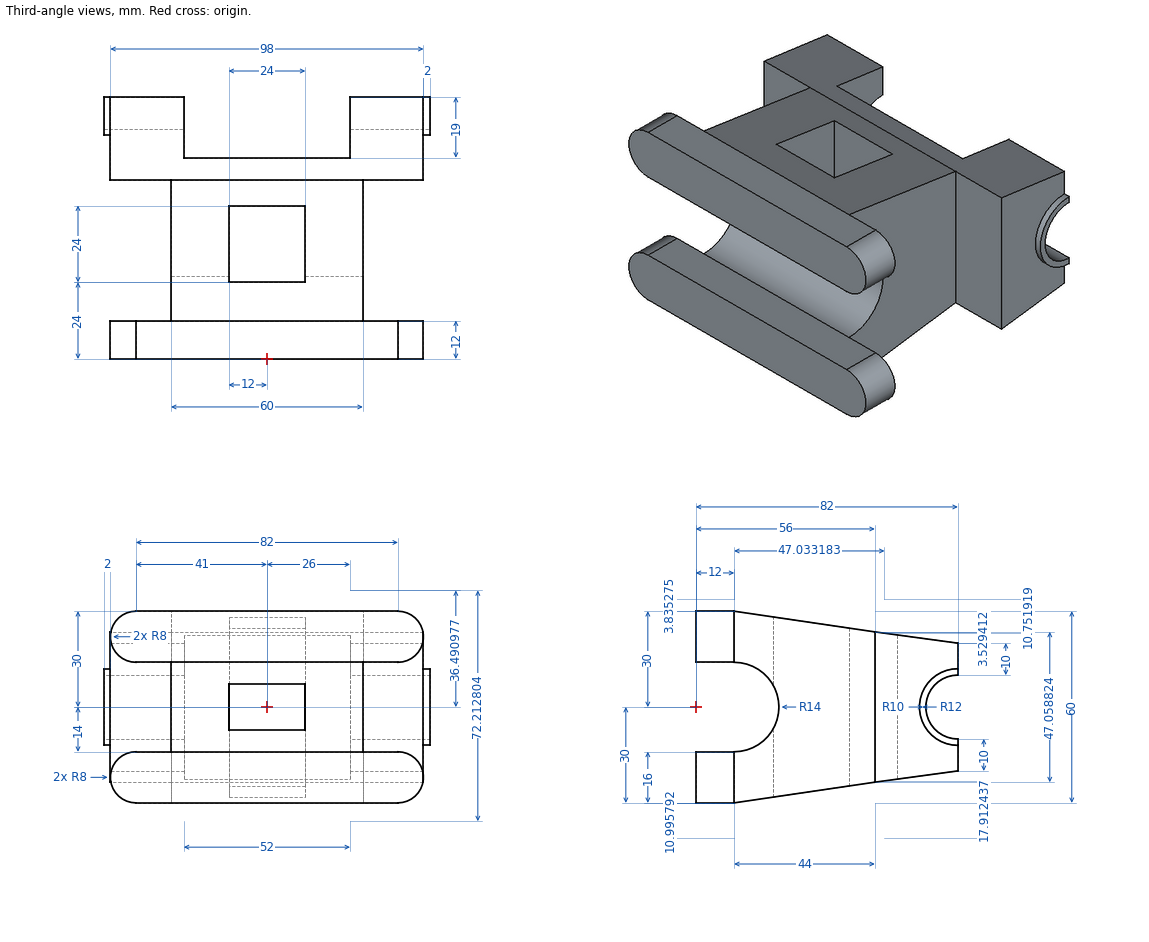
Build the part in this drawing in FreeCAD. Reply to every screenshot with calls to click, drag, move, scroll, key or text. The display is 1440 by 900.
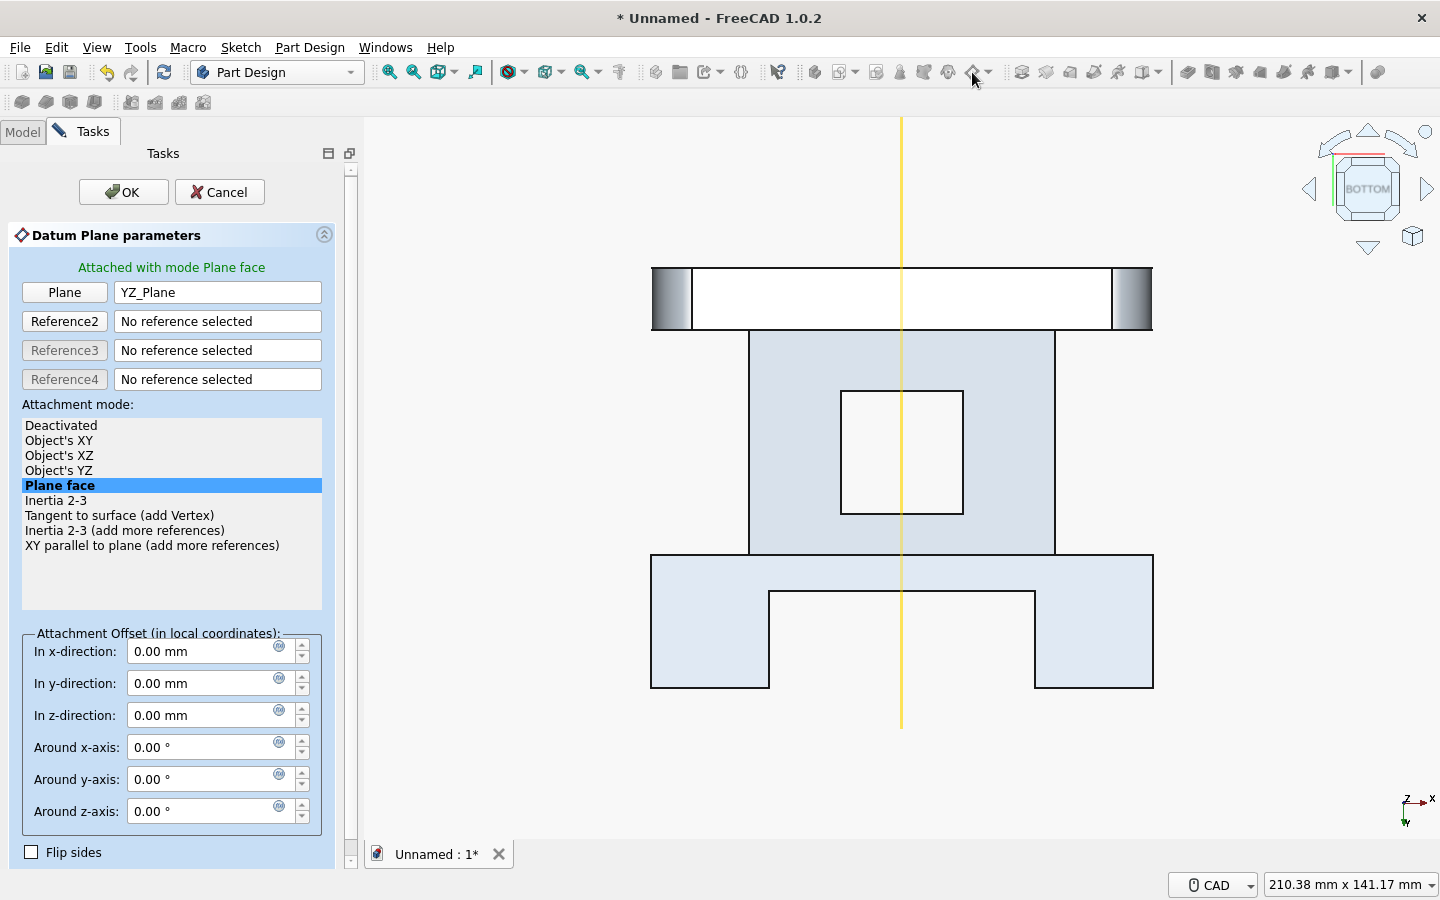
triple_click(210, 715)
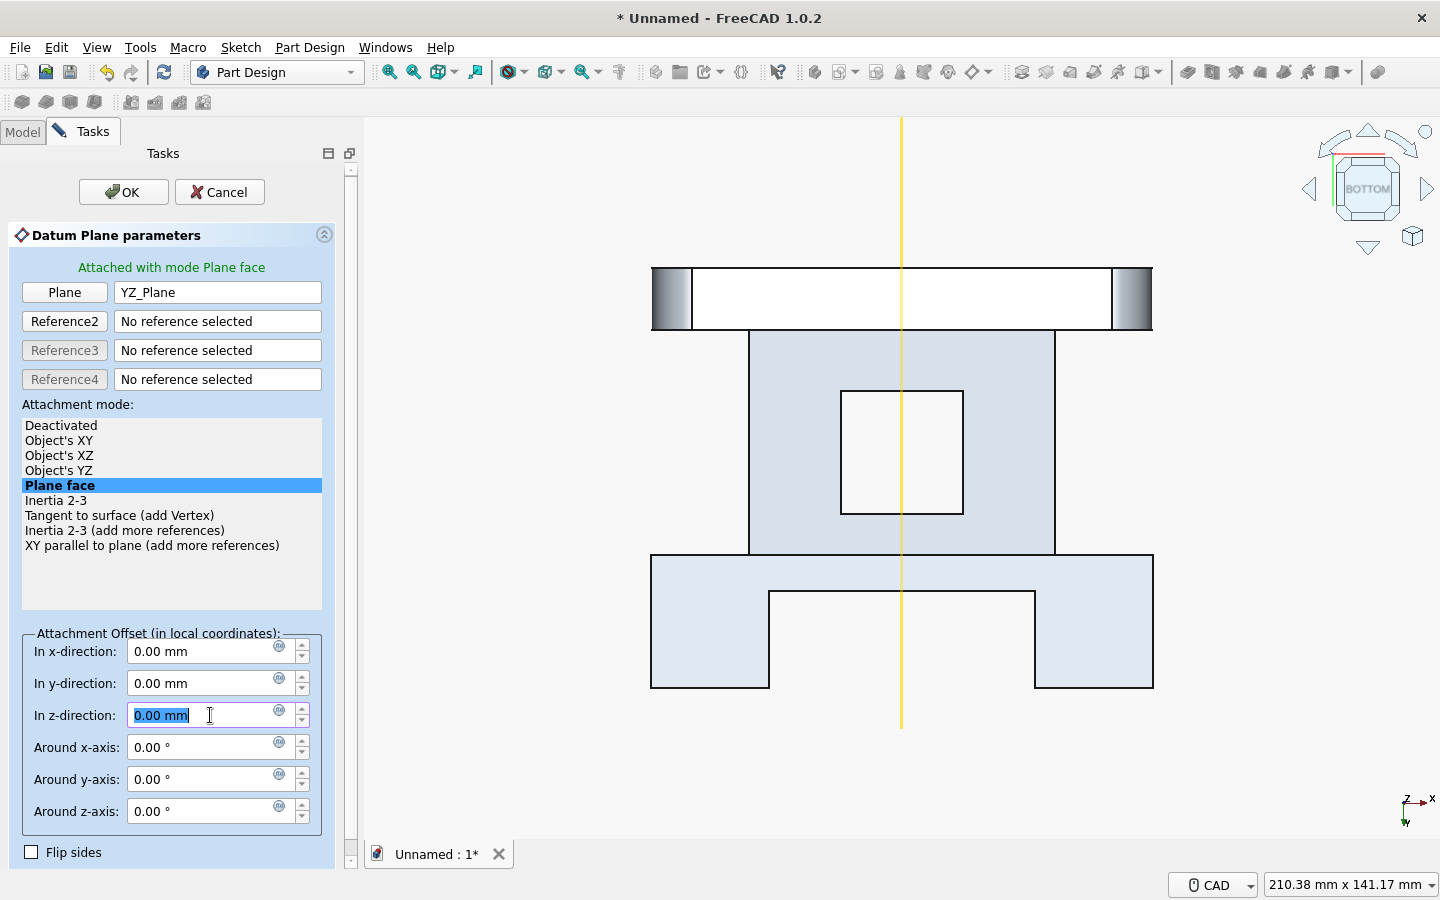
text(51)
key(Tab)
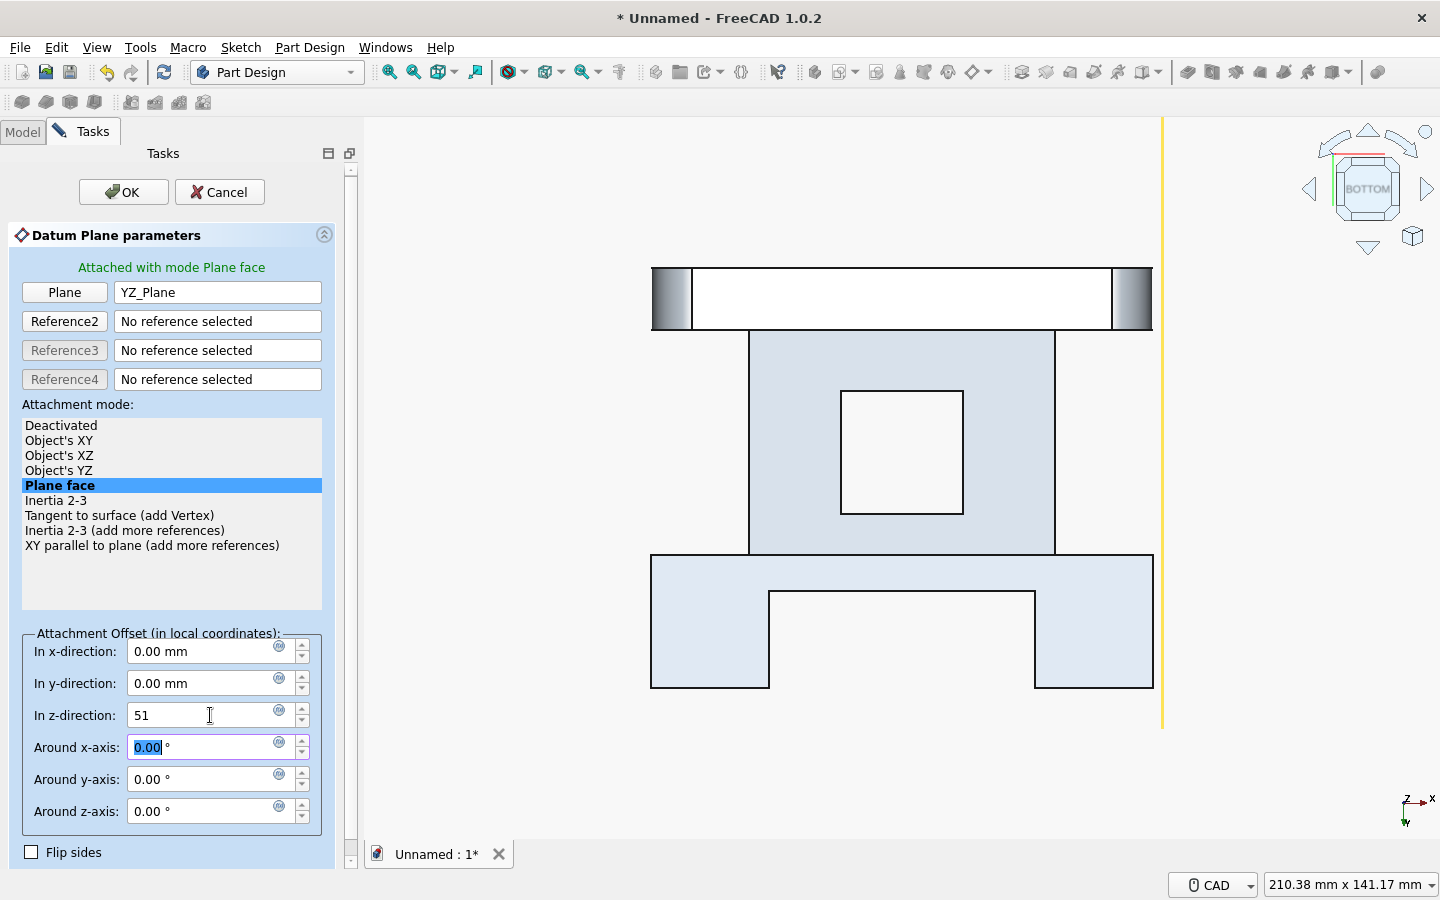
click(124, 192)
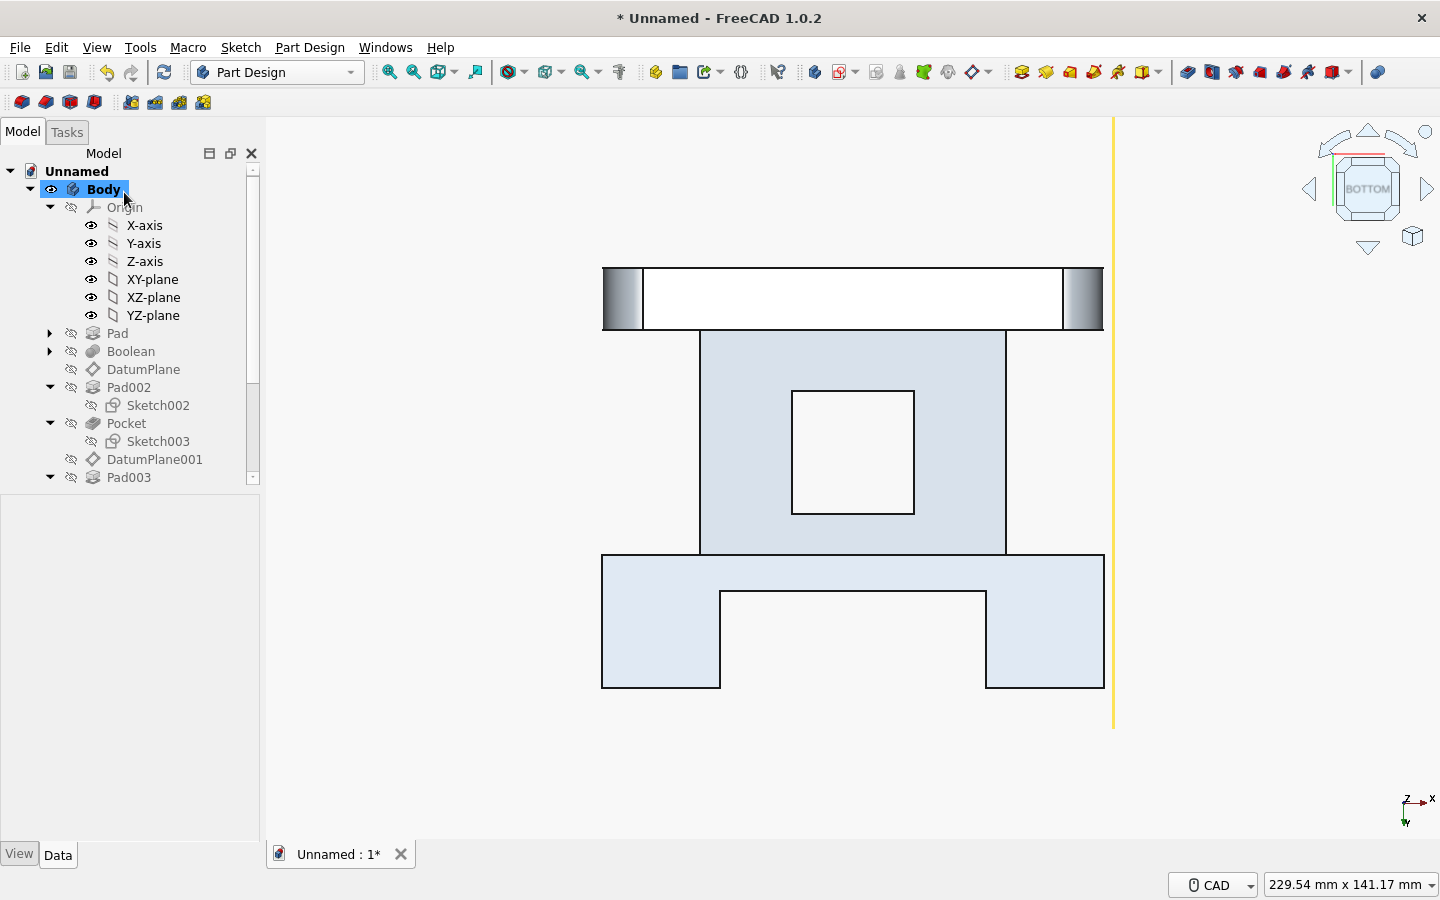
scroll(100, 329, down, 3)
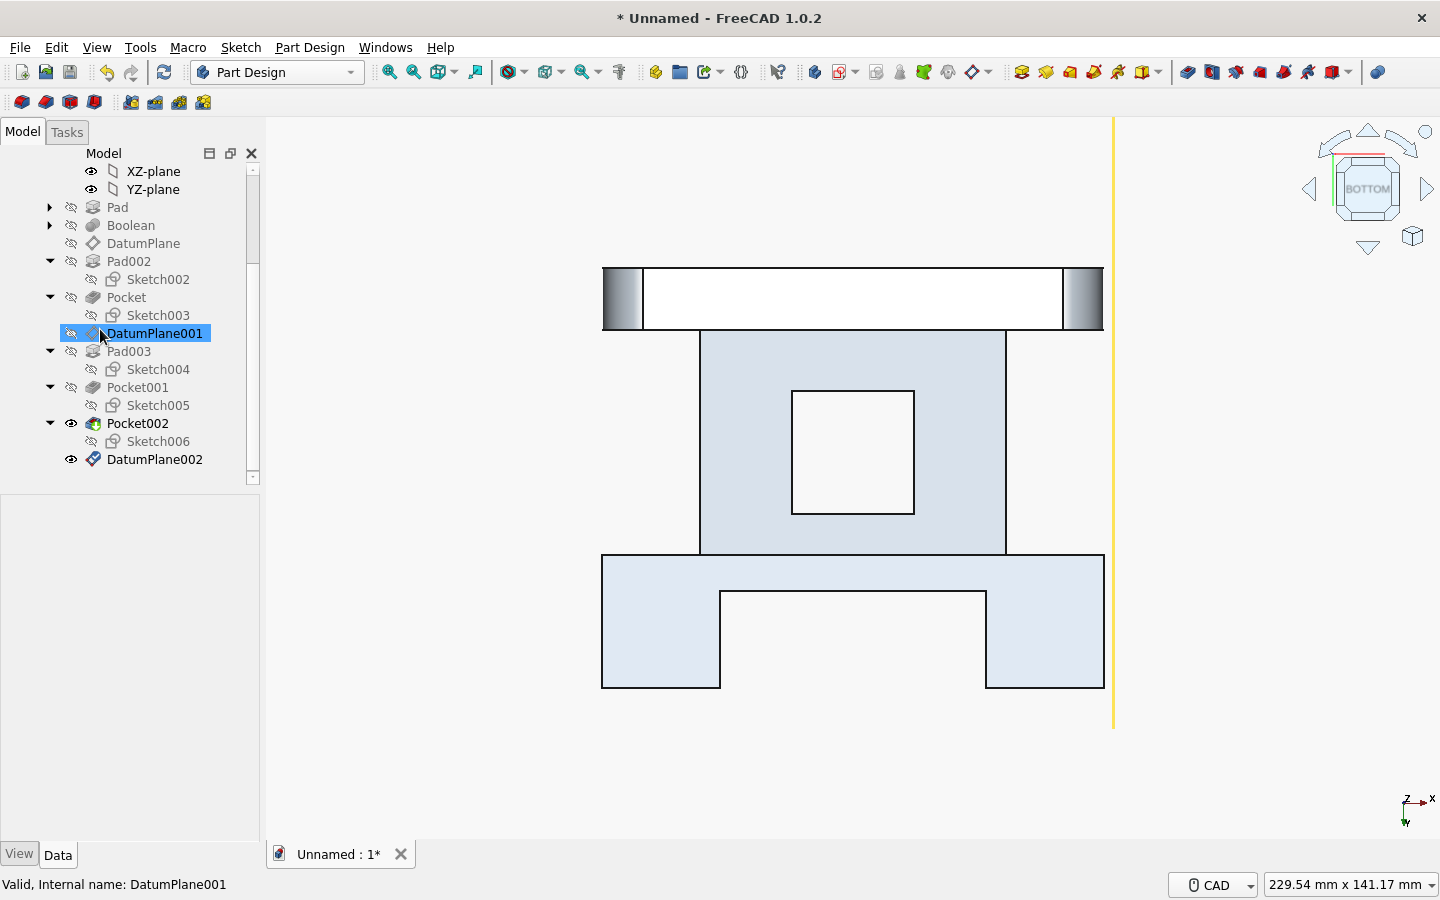
click(116, 459)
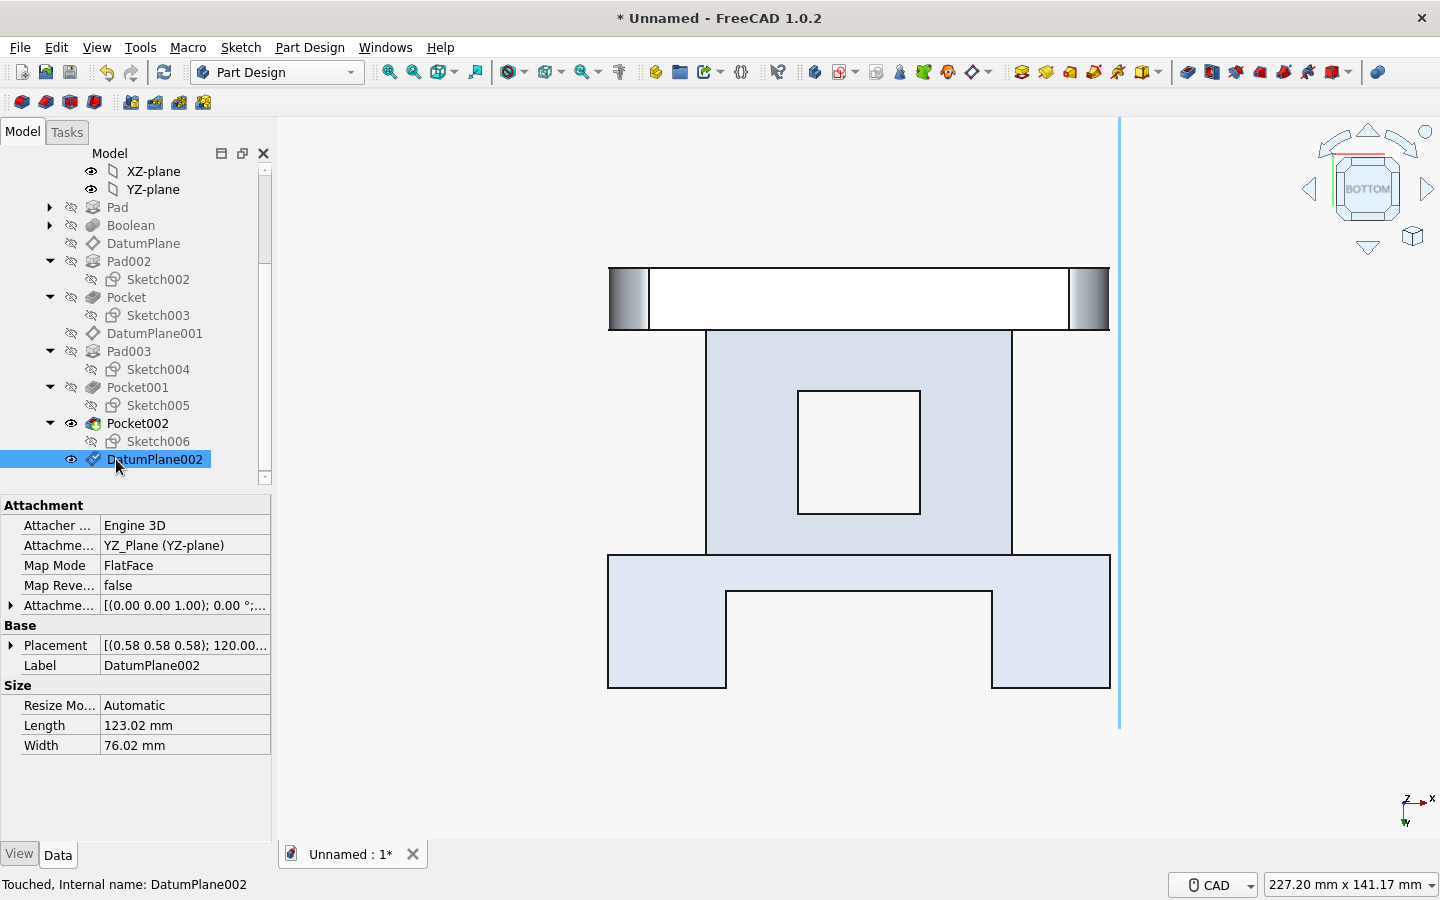
click(840, 72)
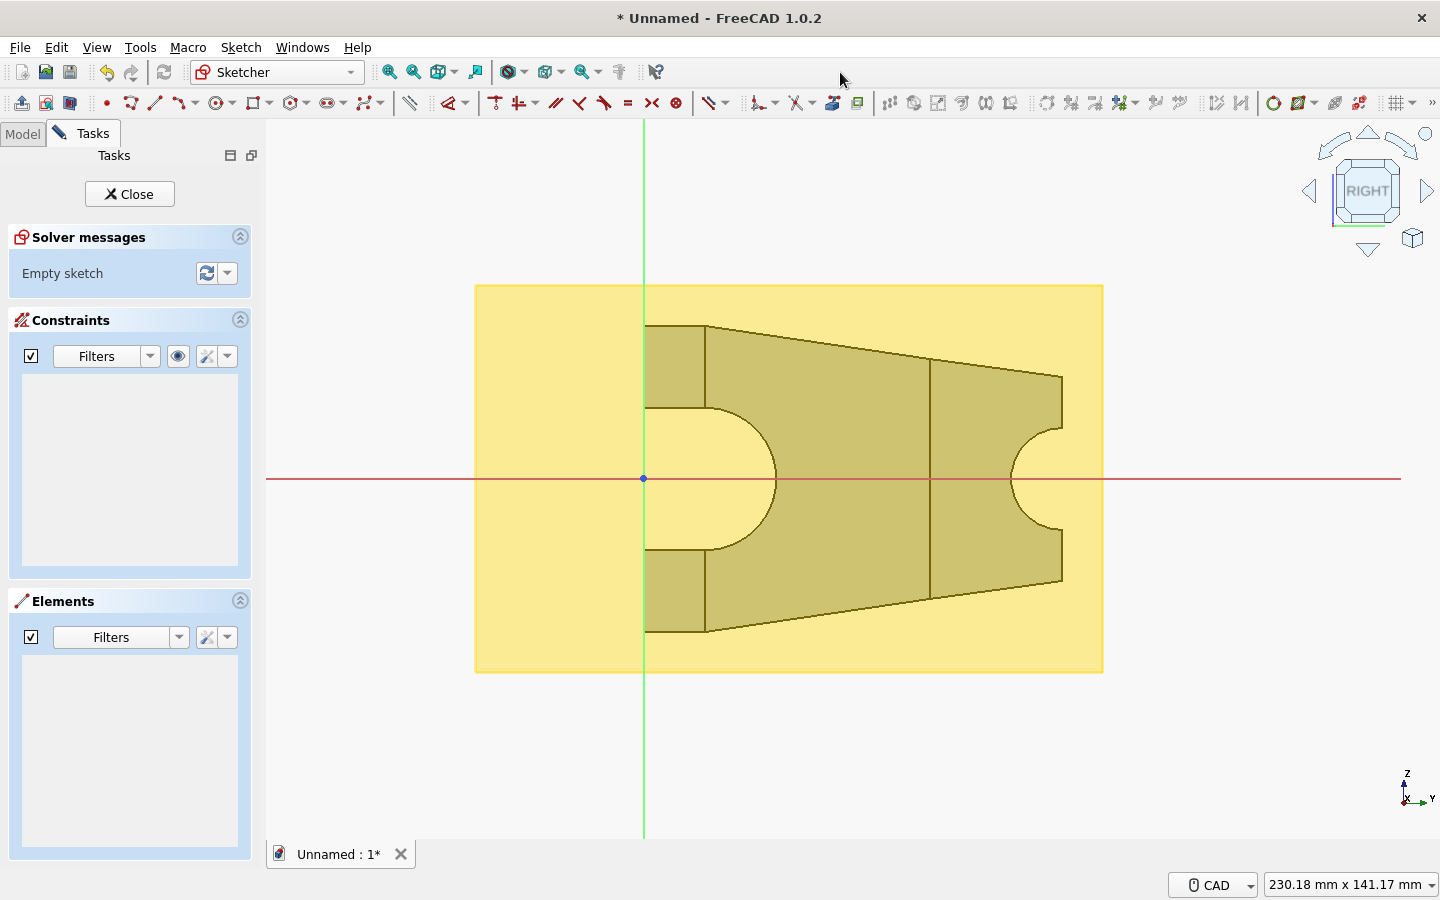
scroll(1112, 479, up, 7)